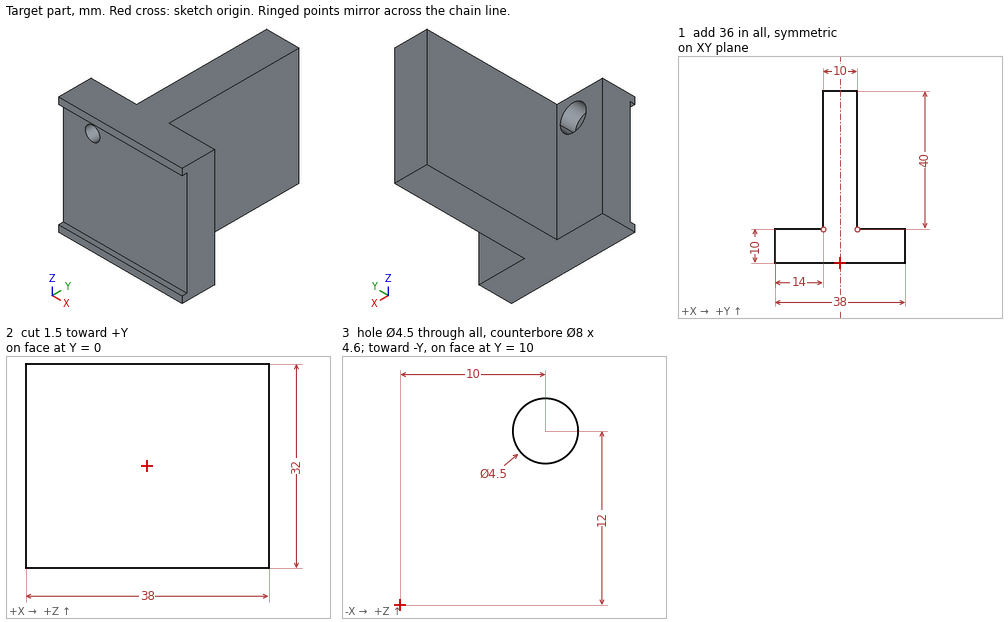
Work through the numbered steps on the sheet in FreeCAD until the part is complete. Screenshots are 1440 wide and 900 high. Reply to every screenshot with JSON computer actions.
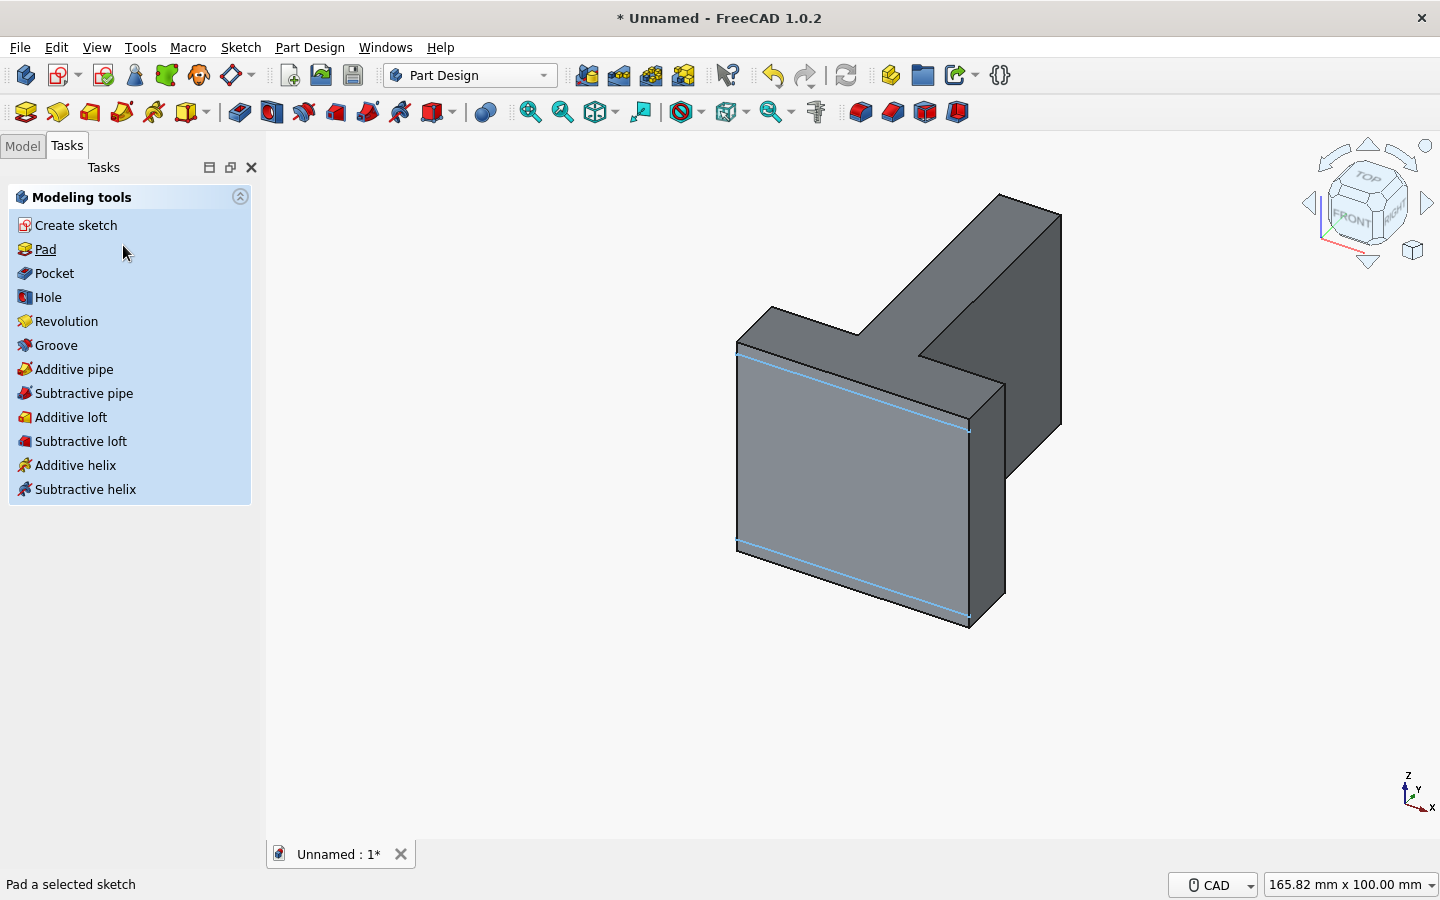
{"action": "left_click", "coordinate": [240, 112]}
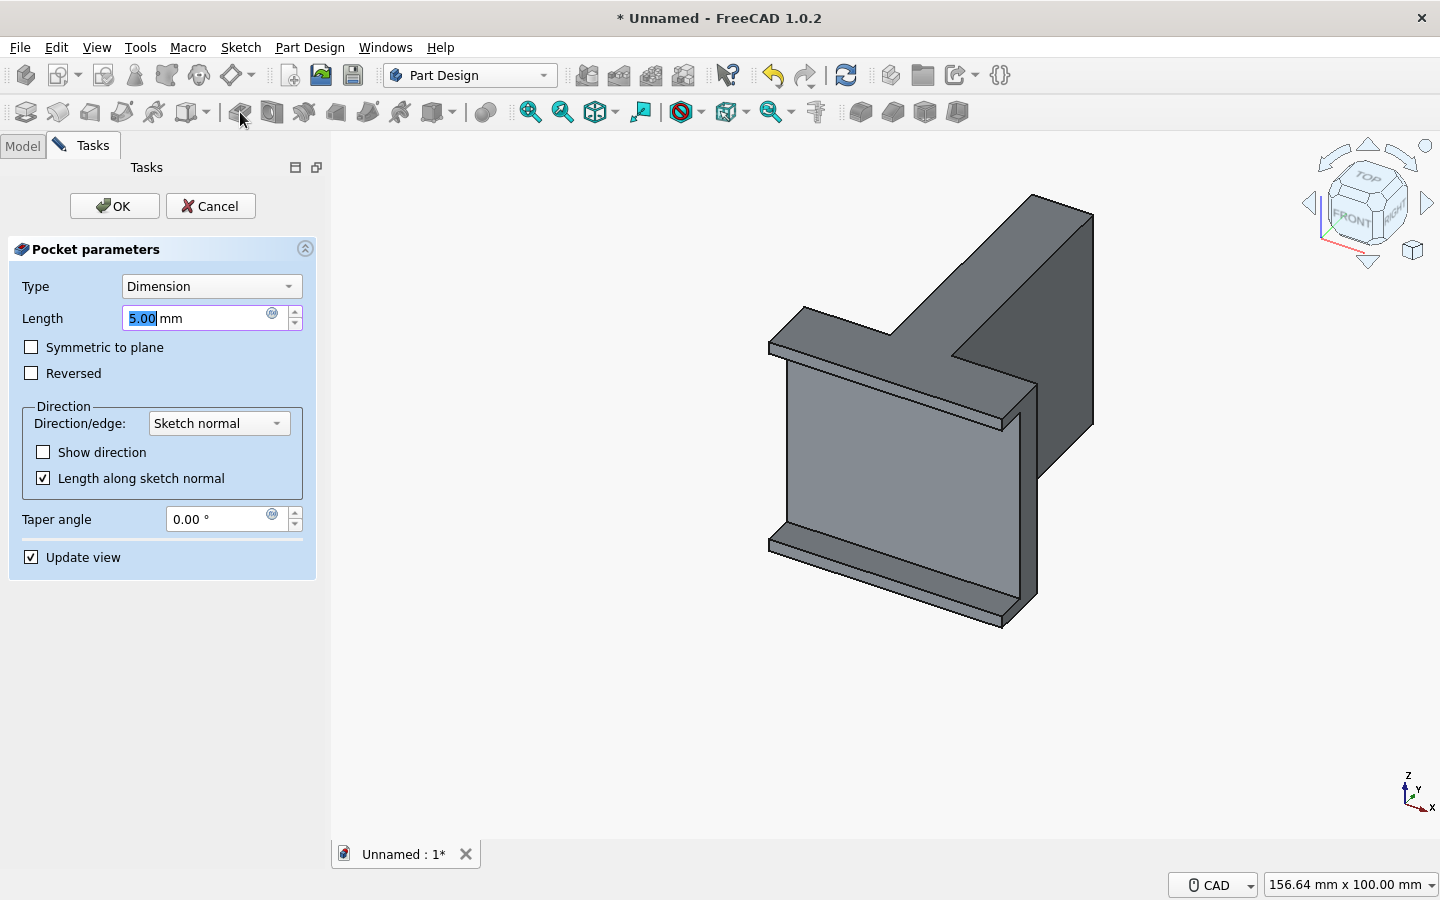
{"action": "type", "text": "1.5"}
{"action": "key", "text": "Tab"}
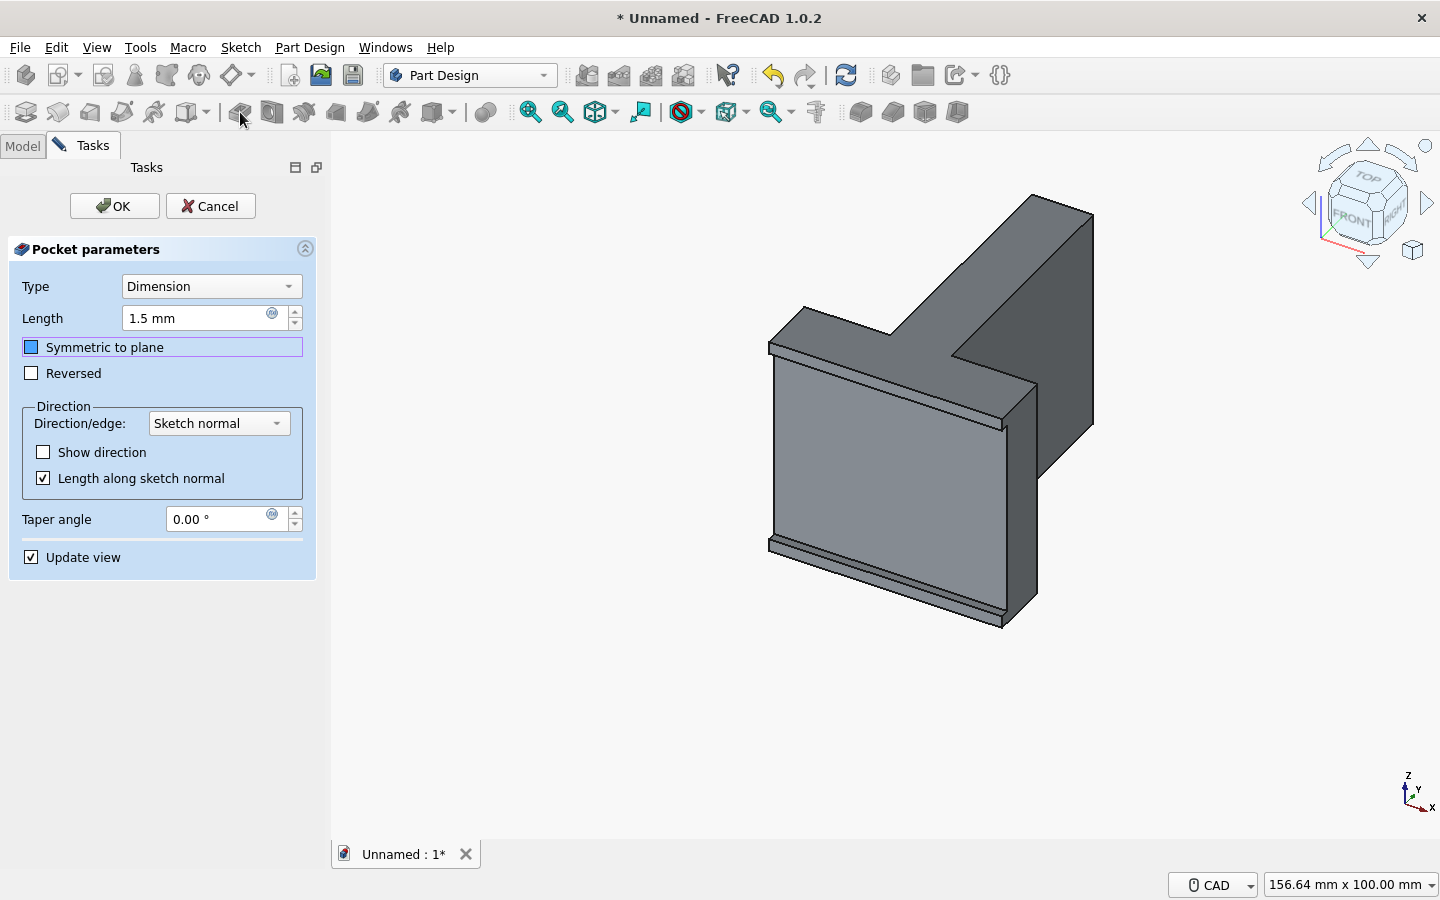
{"action": "left_click", "coordinate": [115, 206]}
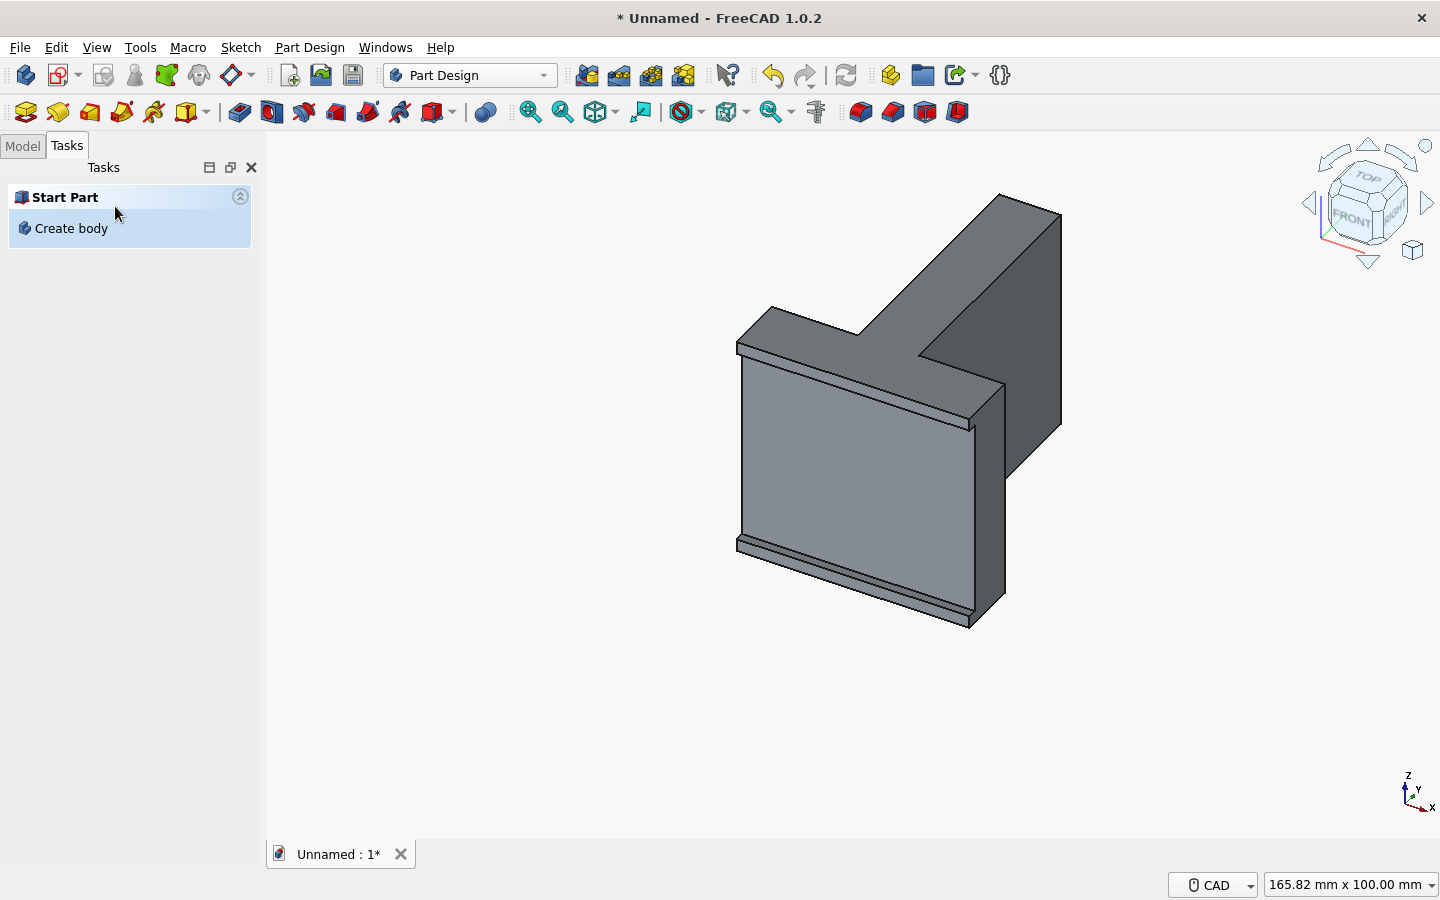
{"action": "key", "text": "4"}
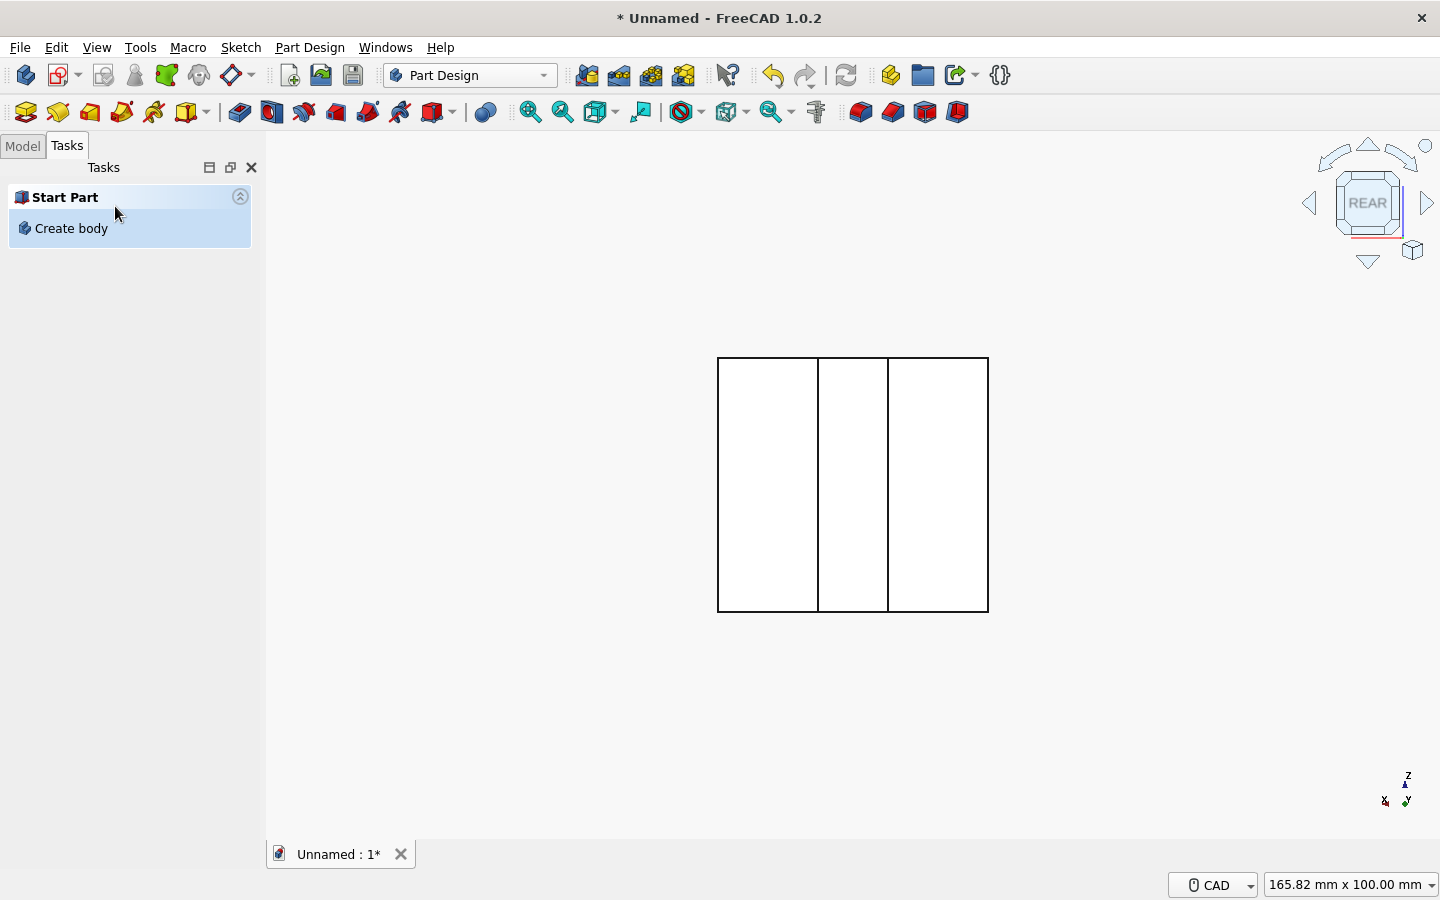
{"action": "left_click", "coordinate": [532, 112]}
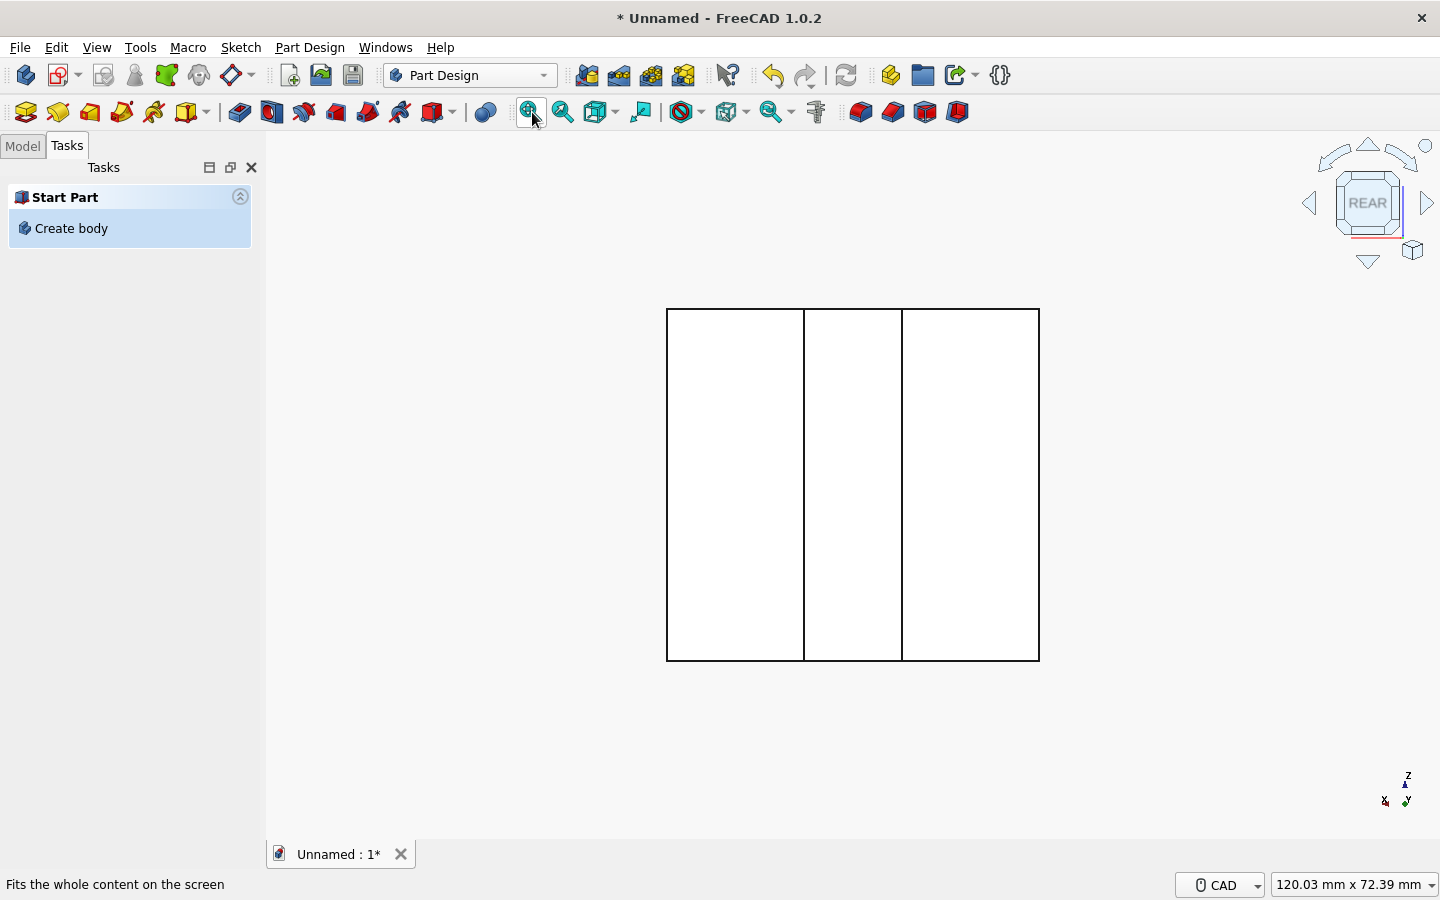
{"action": "left_click", "coordinate": [970, 383]}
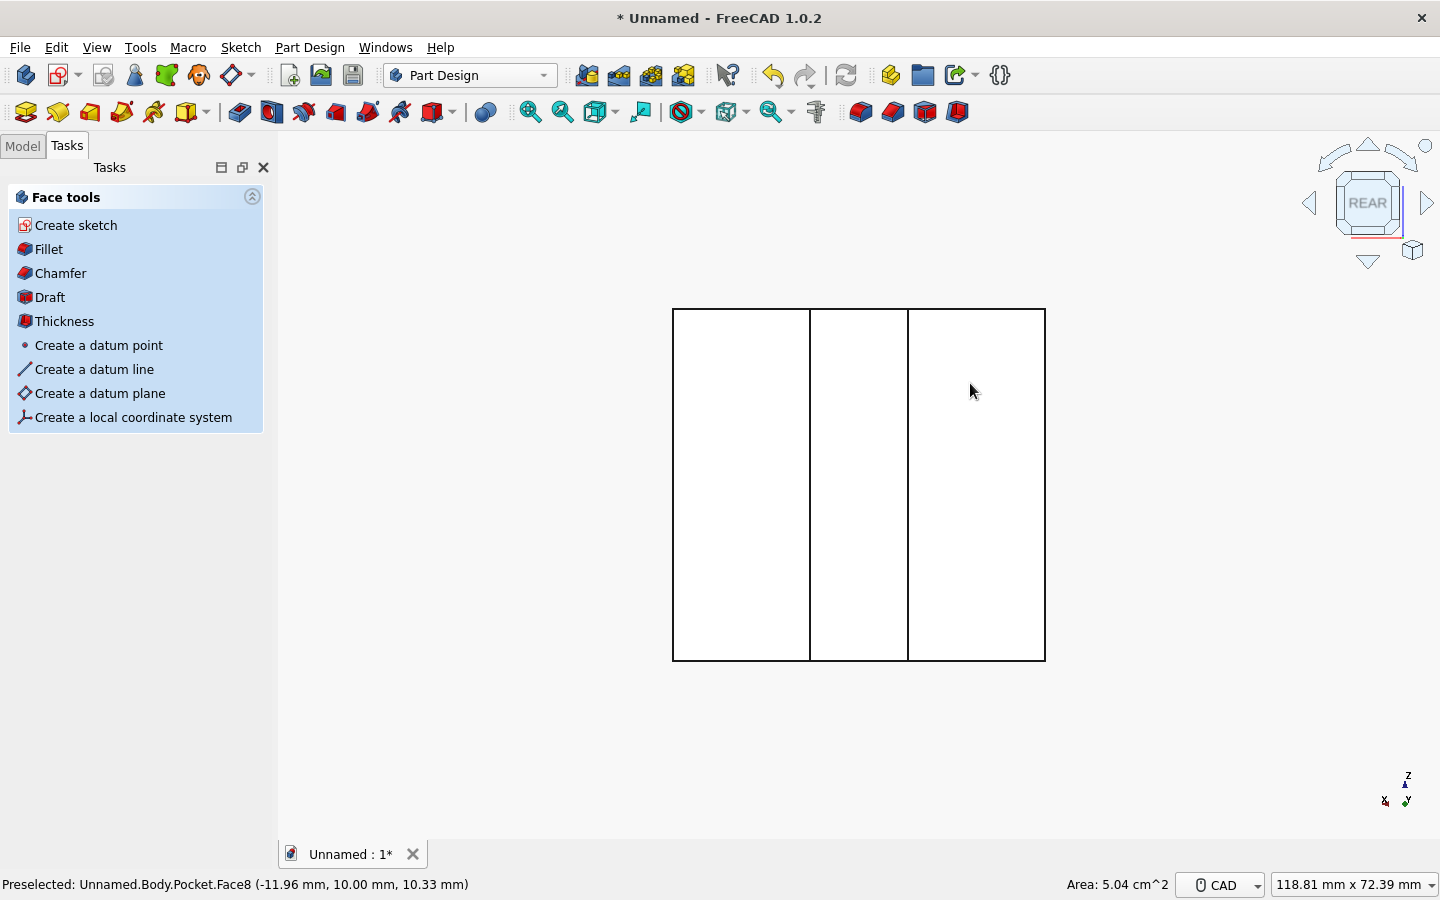
{"action": "left_click", "coordinate": [58, 76]}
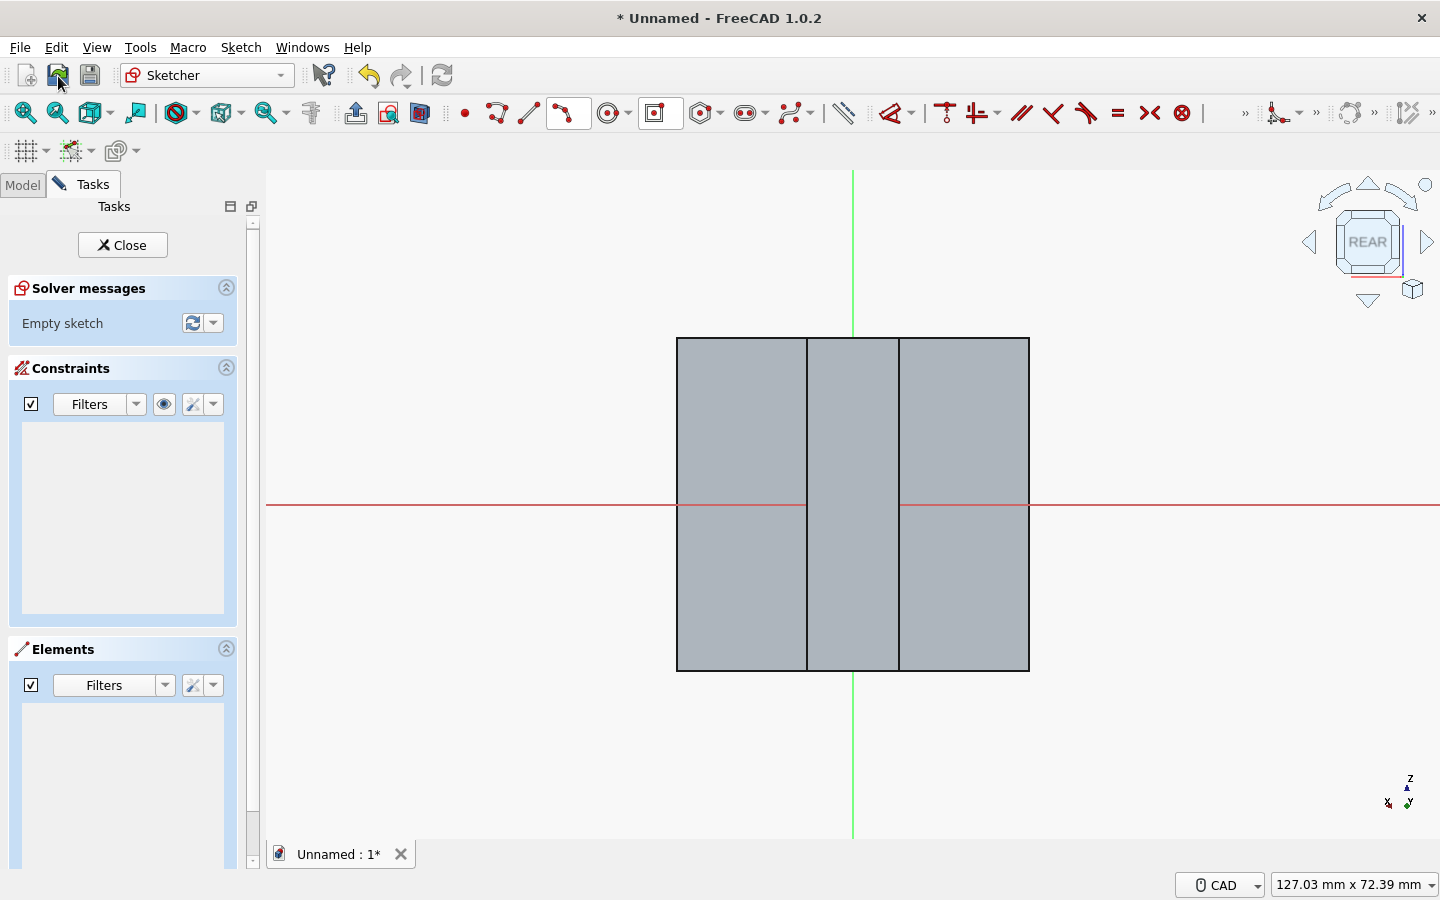
{"action": "left_click", "coordinate": [420, 114]}